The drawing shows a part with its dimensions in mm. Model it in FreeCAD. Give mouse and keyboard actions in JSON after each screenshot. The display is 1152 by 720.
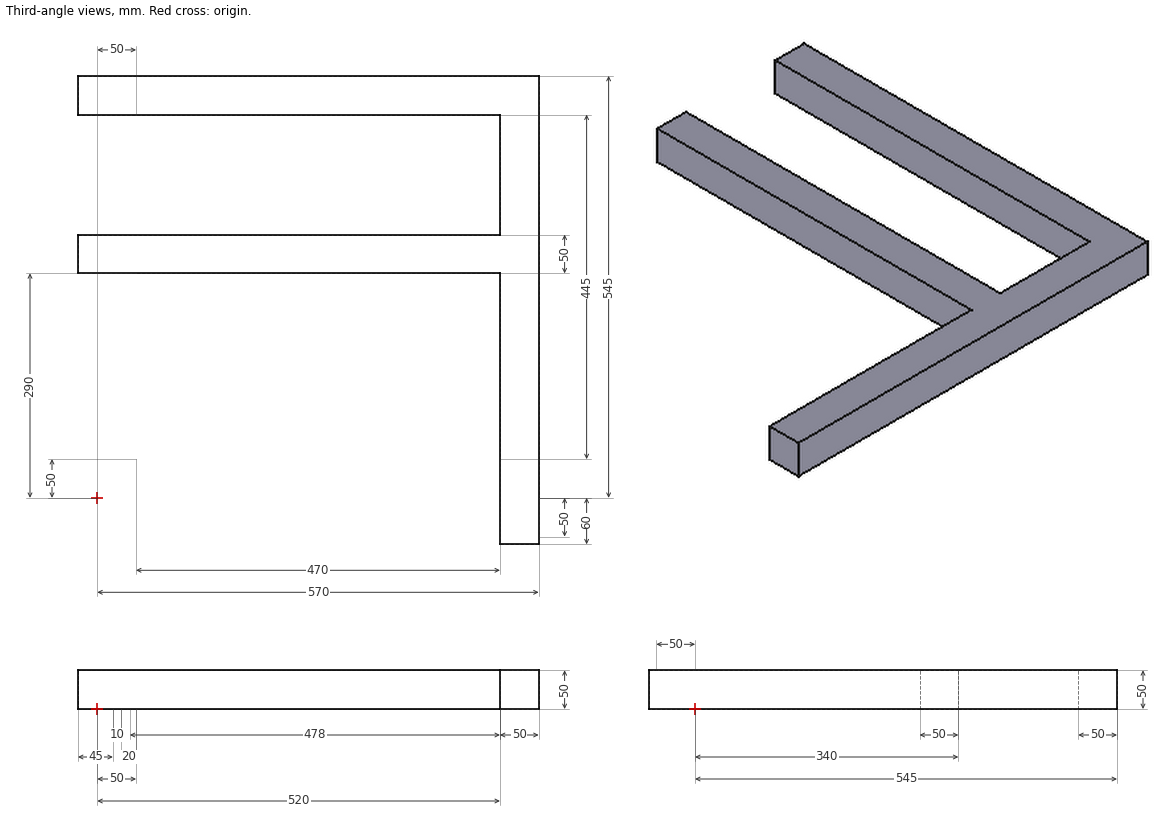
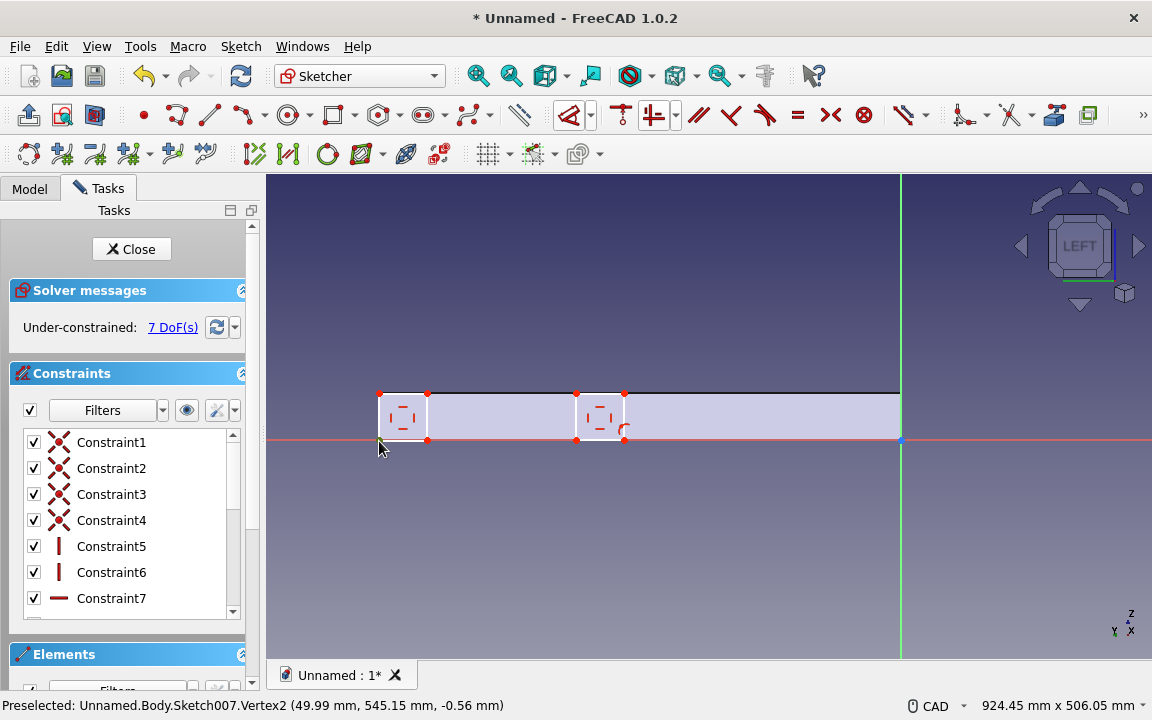
{"action": "left_click", "coordinate": [344, 440]}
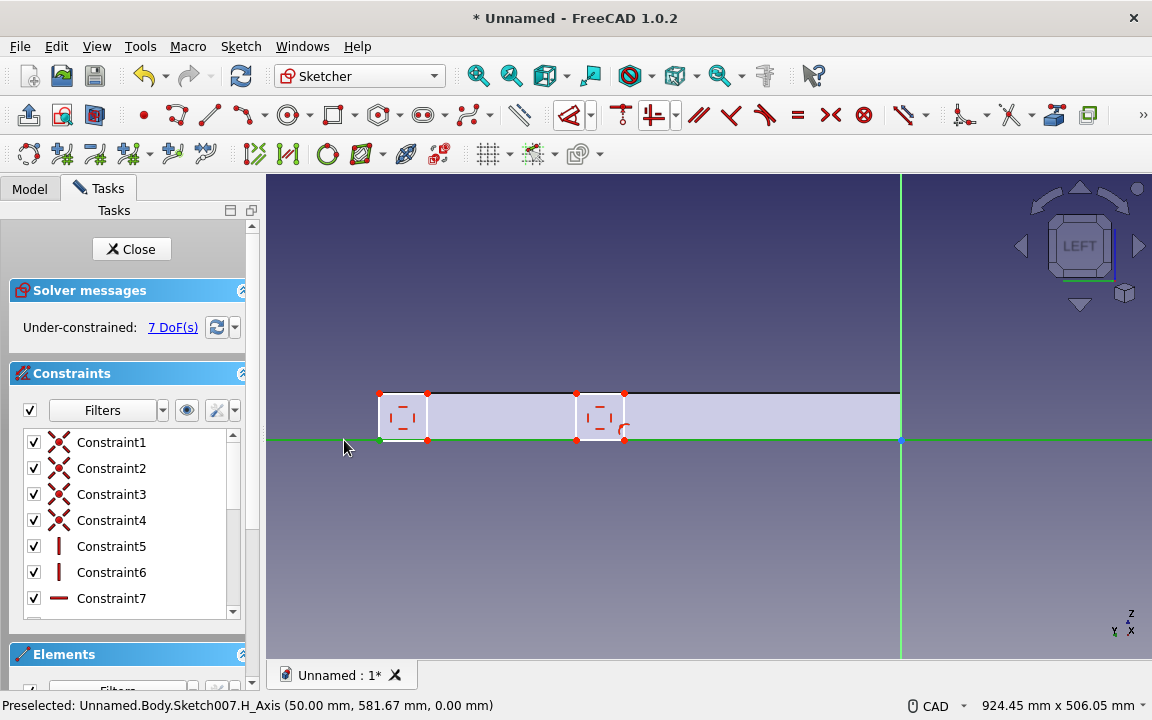
{"action": "key", "text": "c"}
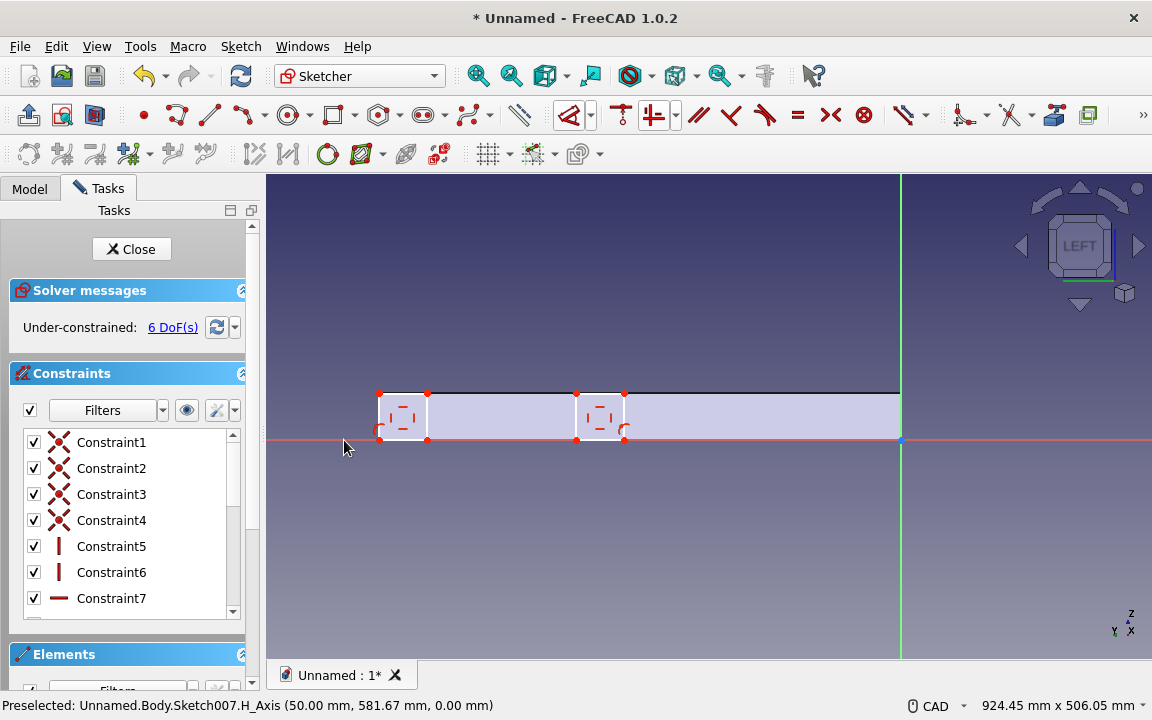
{"action": "left_click", "coordinate": [379, 408]}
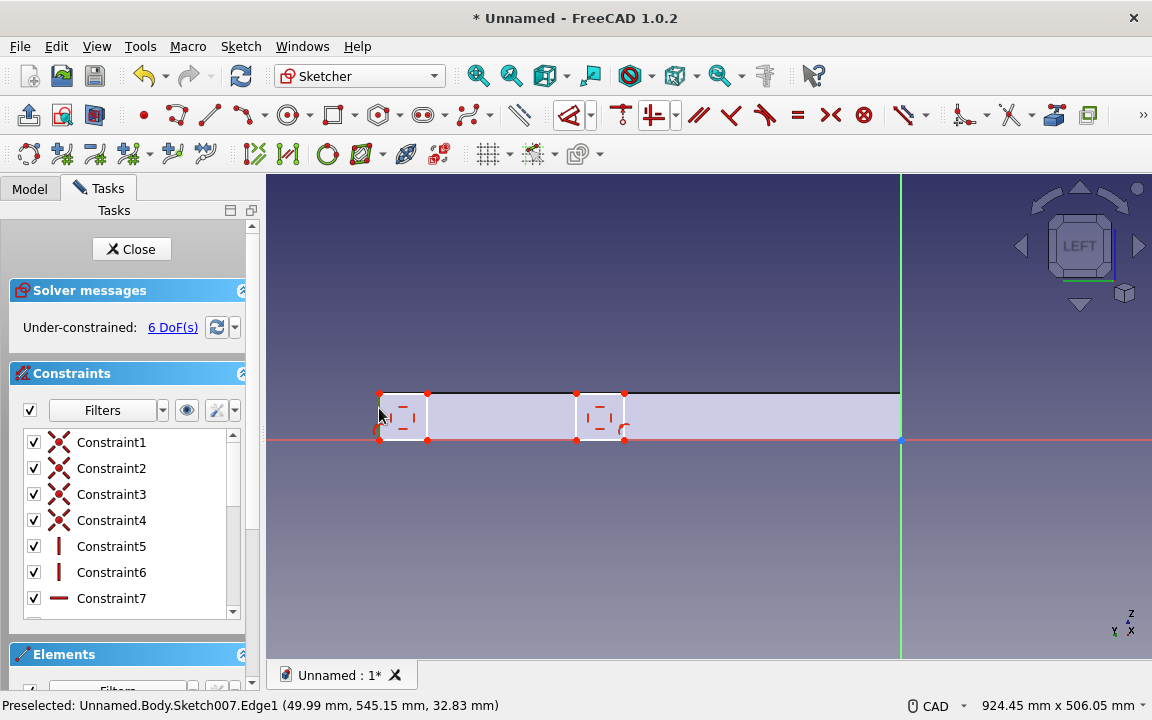
{"action": "key", "text": "i"}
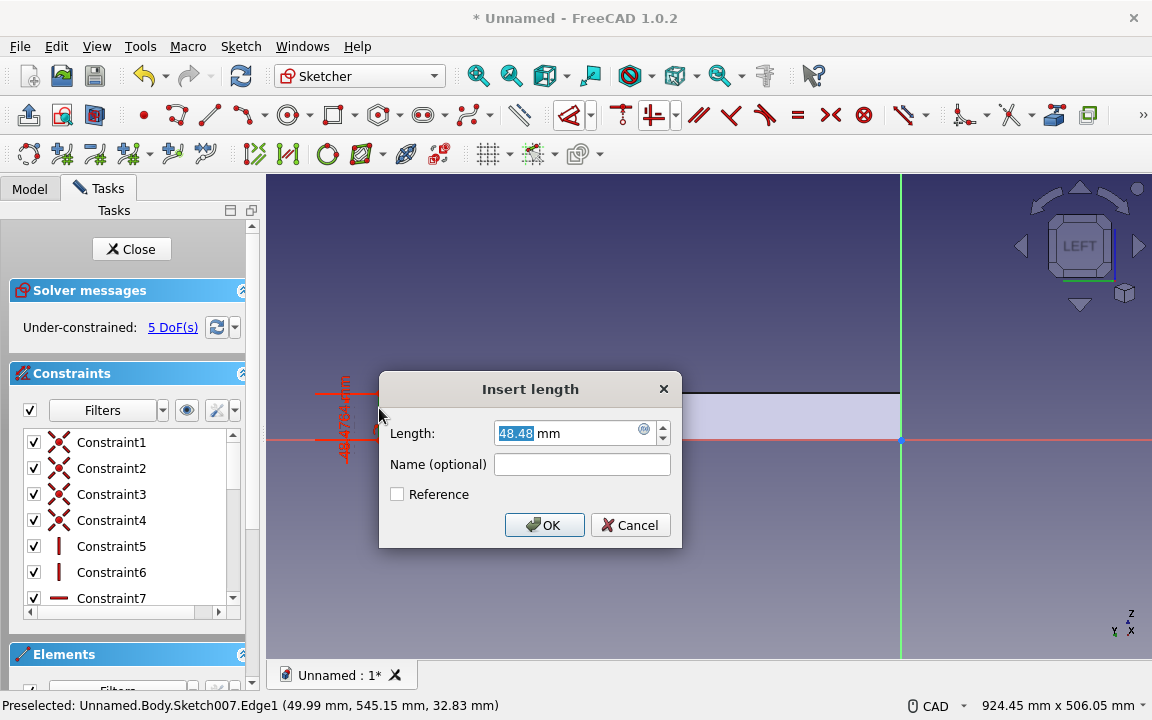
{"action": "type", "text": "50"}
{"action": "key", "text": "Return"}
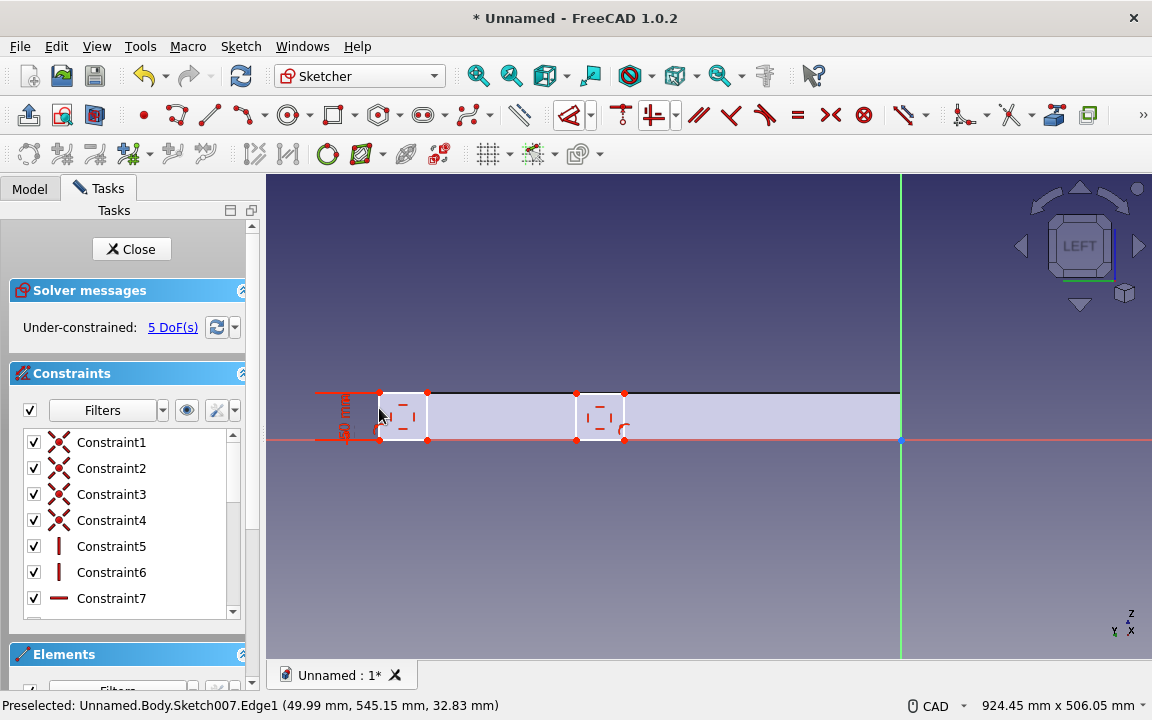
{"action": "left_click", "coordinate": [393, 440]}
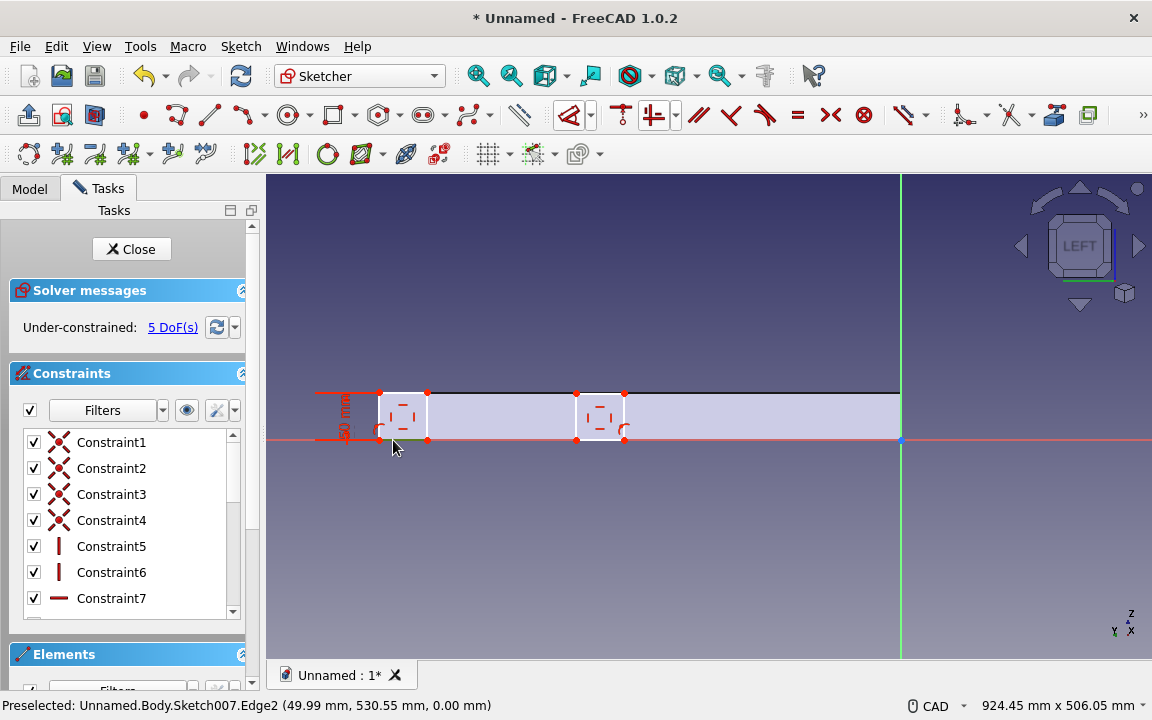
{"action": "key", "text": "l"}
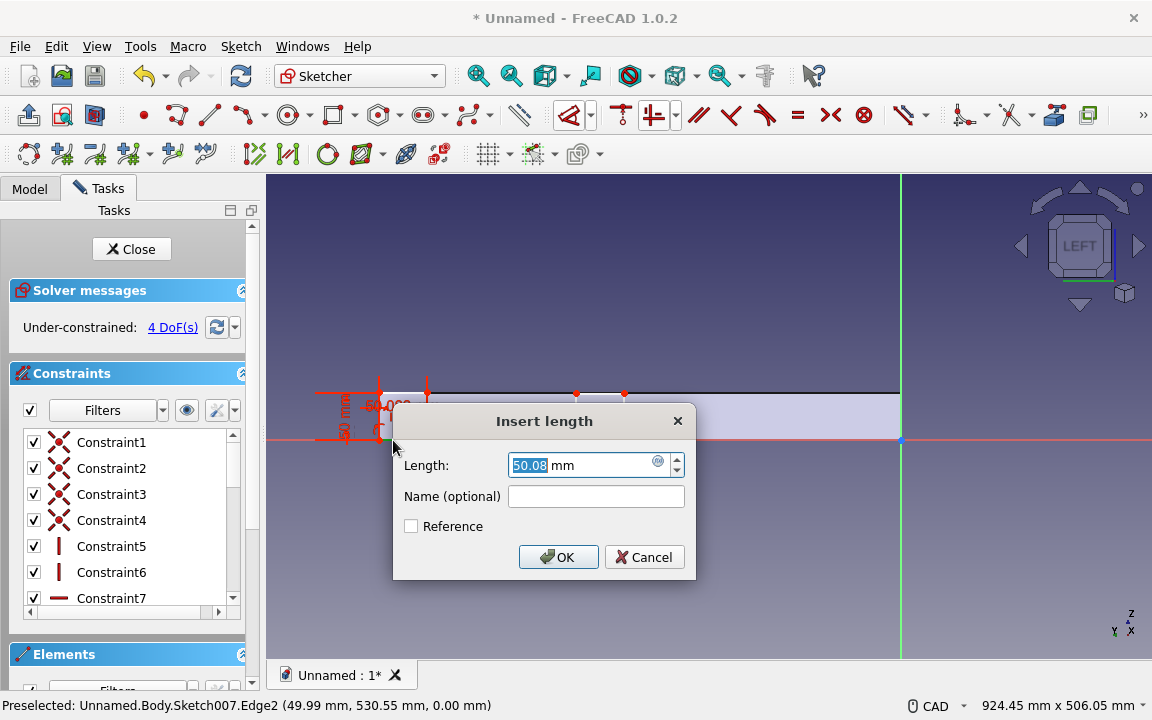
{"action": "type", "text": "50"}
{"action": "key", "text": "Return"}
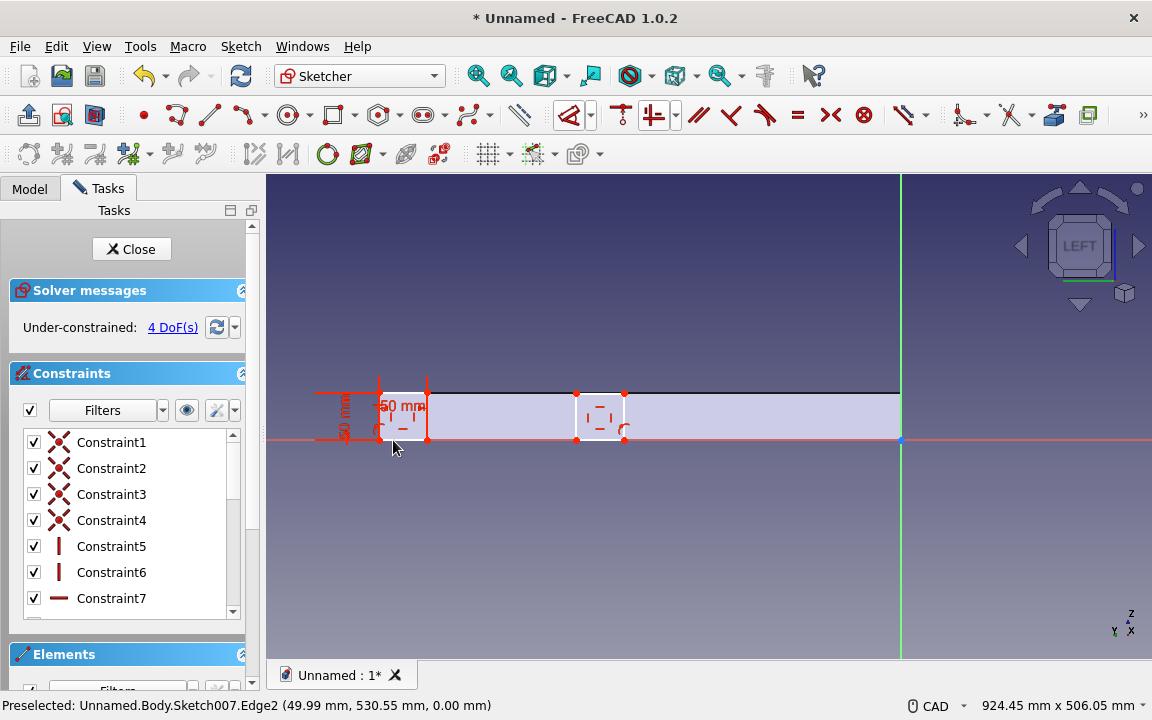
{"action": "left_click", "coordinate": [576, 408]}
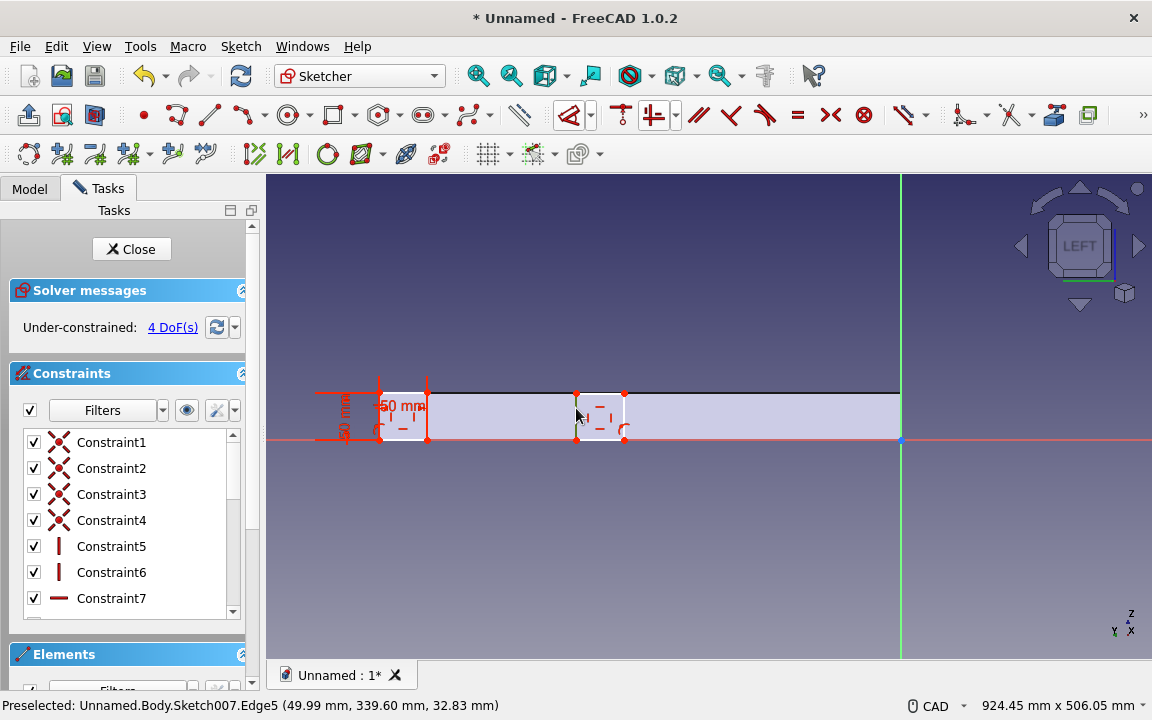
{"action": "key", "text": "i"}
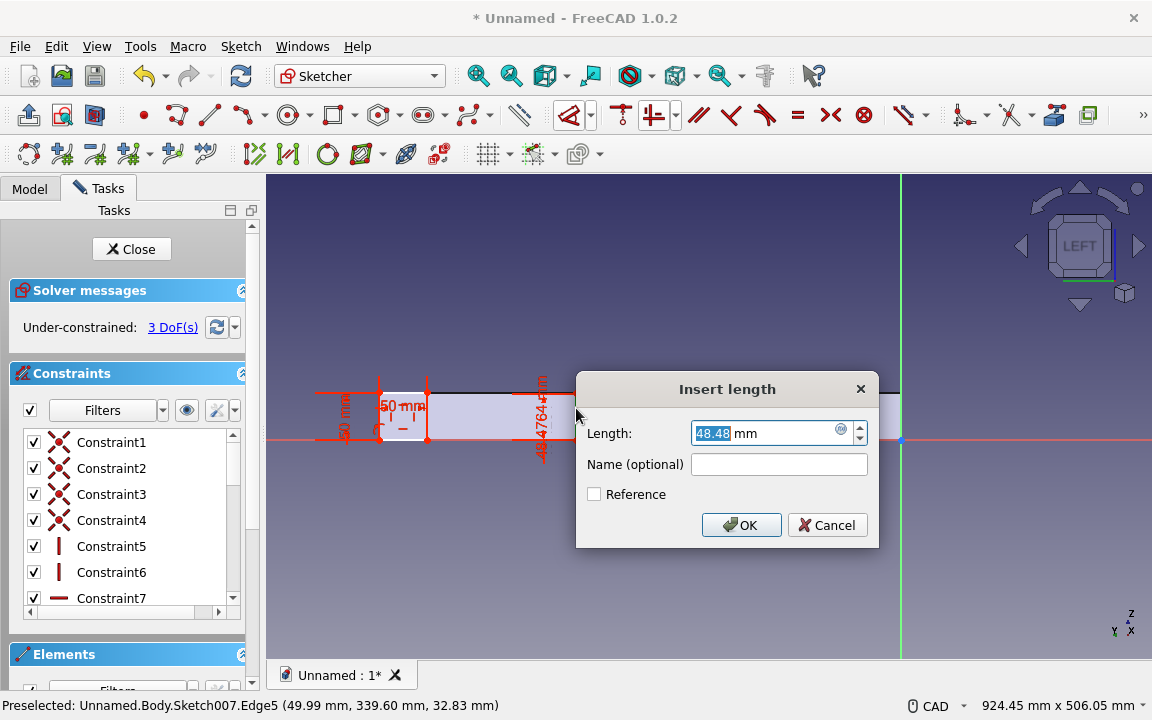
{"action": "type", "text": "50"}
{"action": "key", "text": "Return"}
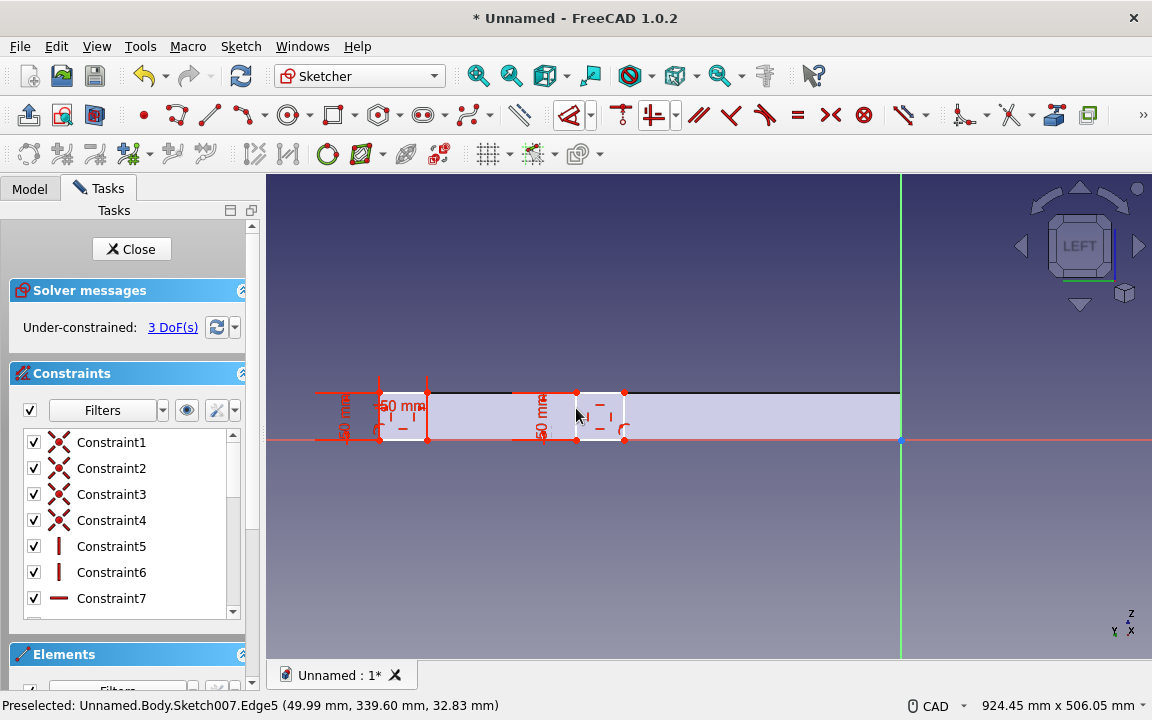
{"action": "left_click", "coordinate": [590, 440]}